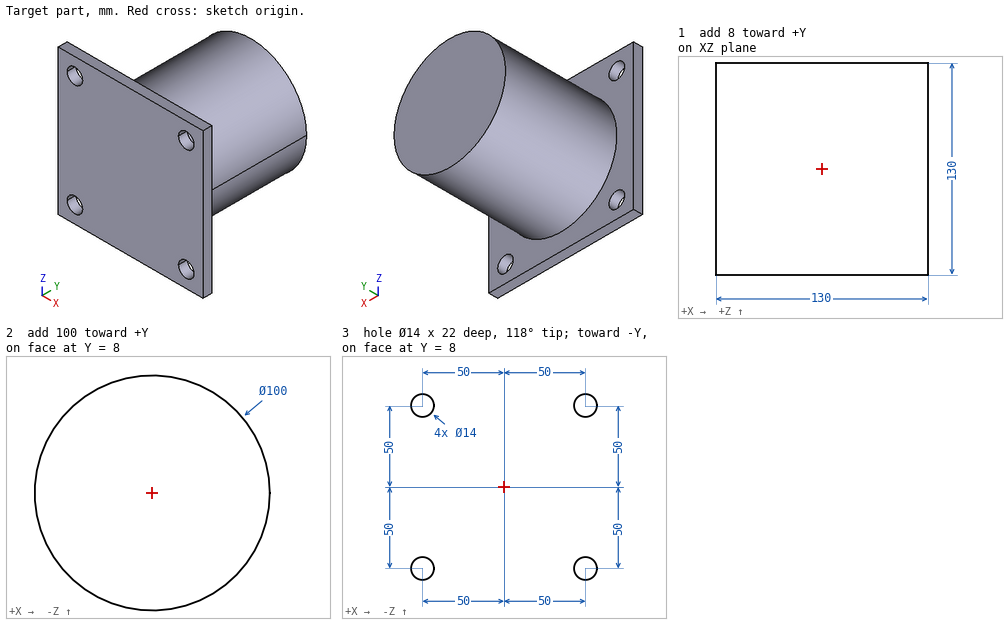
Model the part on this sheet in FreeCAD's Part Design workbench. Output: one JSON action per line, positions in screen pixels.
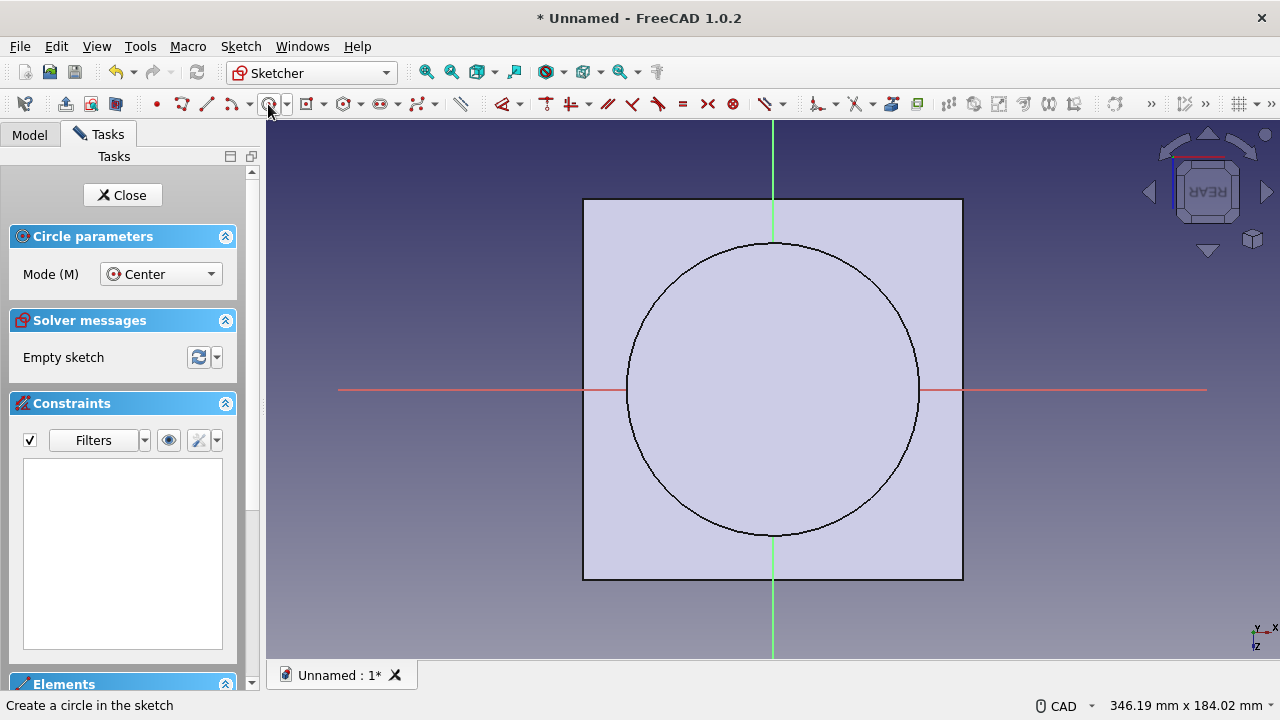
{"action": "left_click", "coordinate": [627, 243]}
{"action": "left_click", "coordinate": [641, 229]}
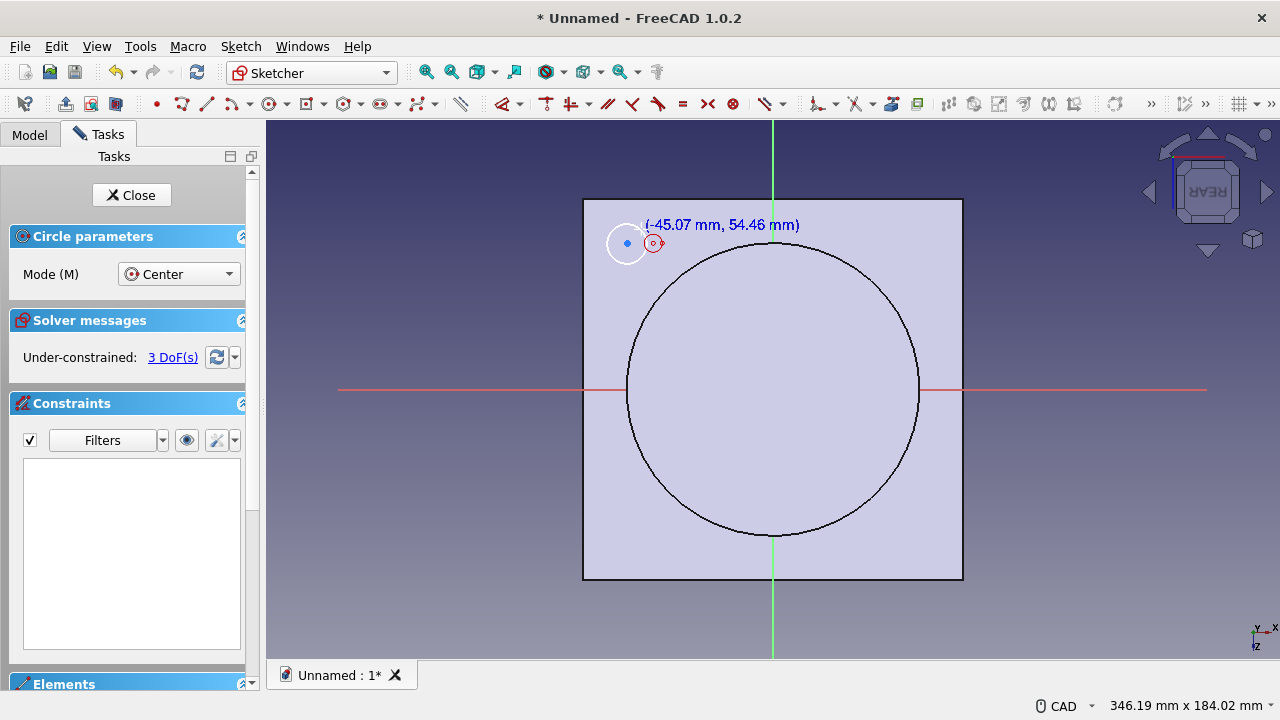
{"action": "left_click", "coordinate": [919, 243]}
{"action": "left_click", "coordinate": [934, 229]}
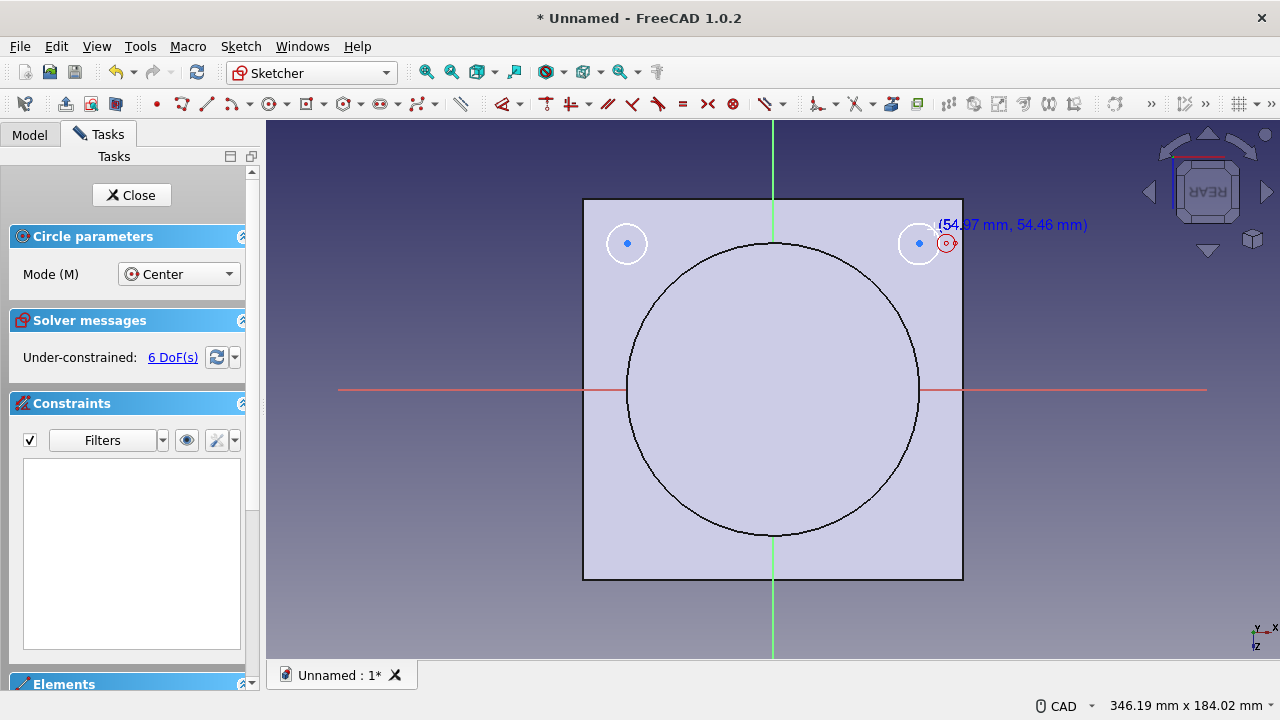
{"action": "left_click", "coordinate": [919, 536]}
{"action": "left_click", "coordinate": [934, 521]}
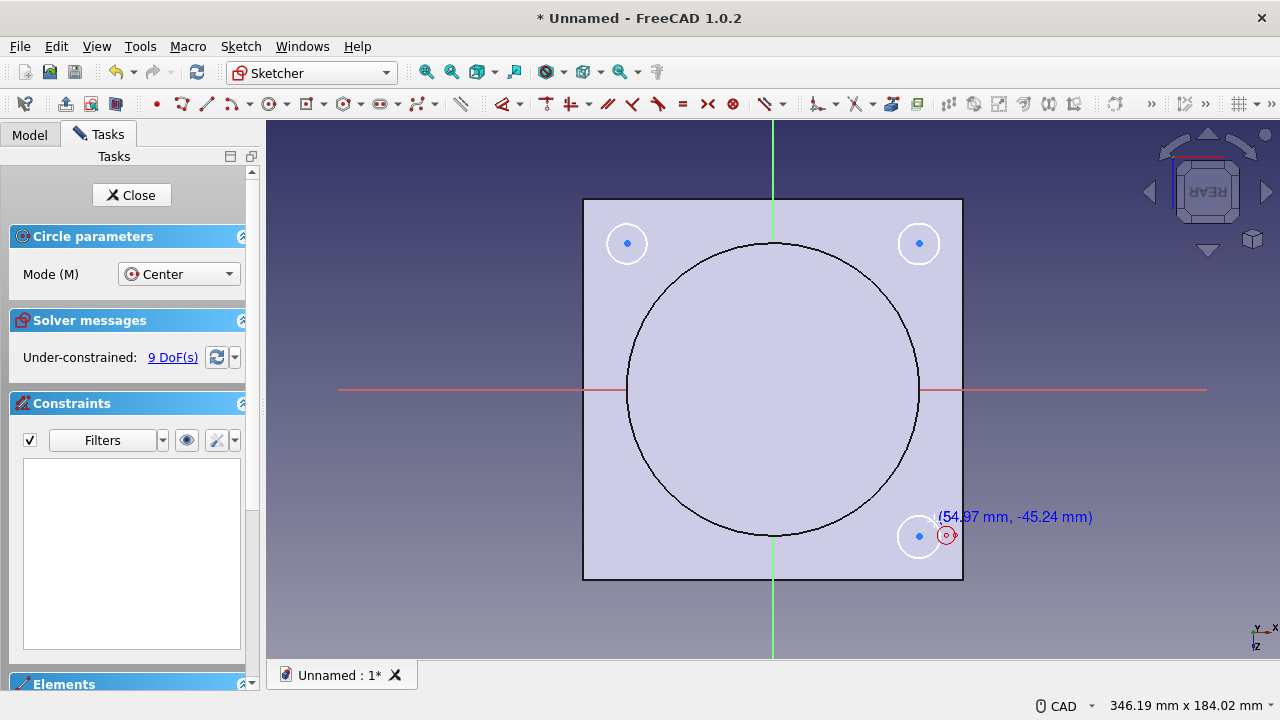
{"action": "left_click", "coordinate": [627, 536]}
{"action": "left_click", "coordinate": [641, 521]}
{"action": "key", "text": "Escape"}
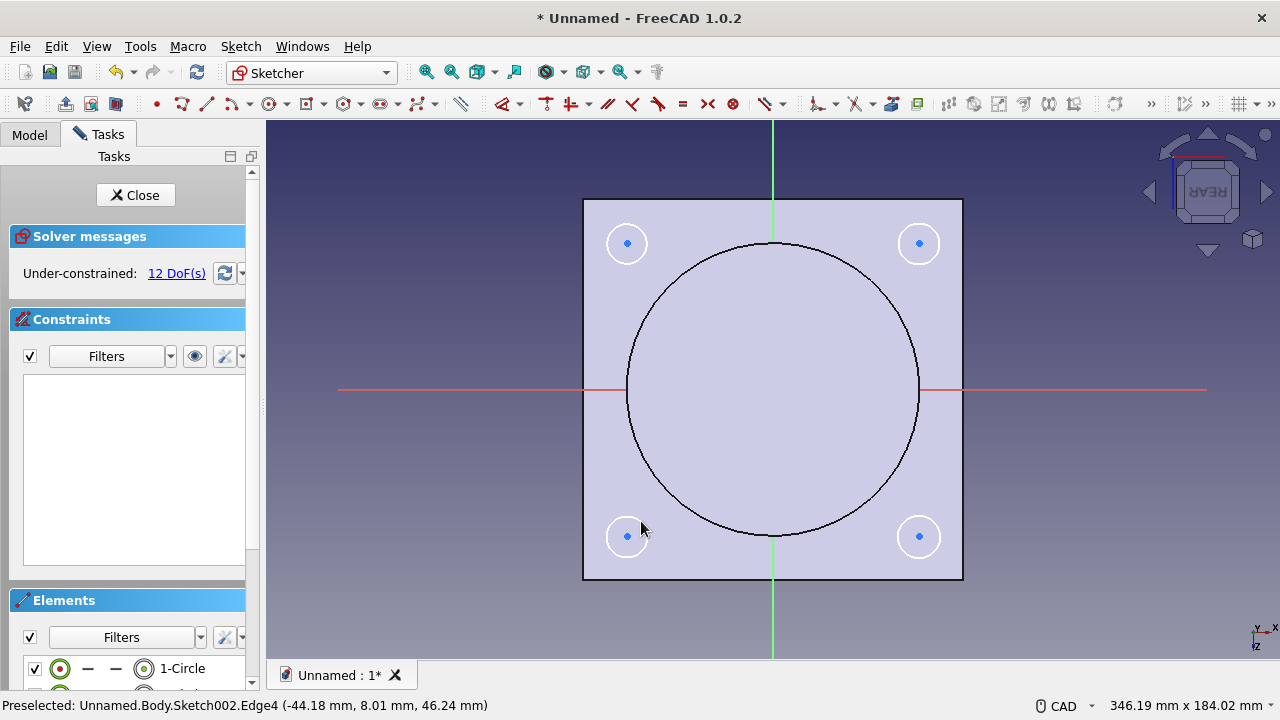
{"action": "left_click", "coordinate": [641, 230]}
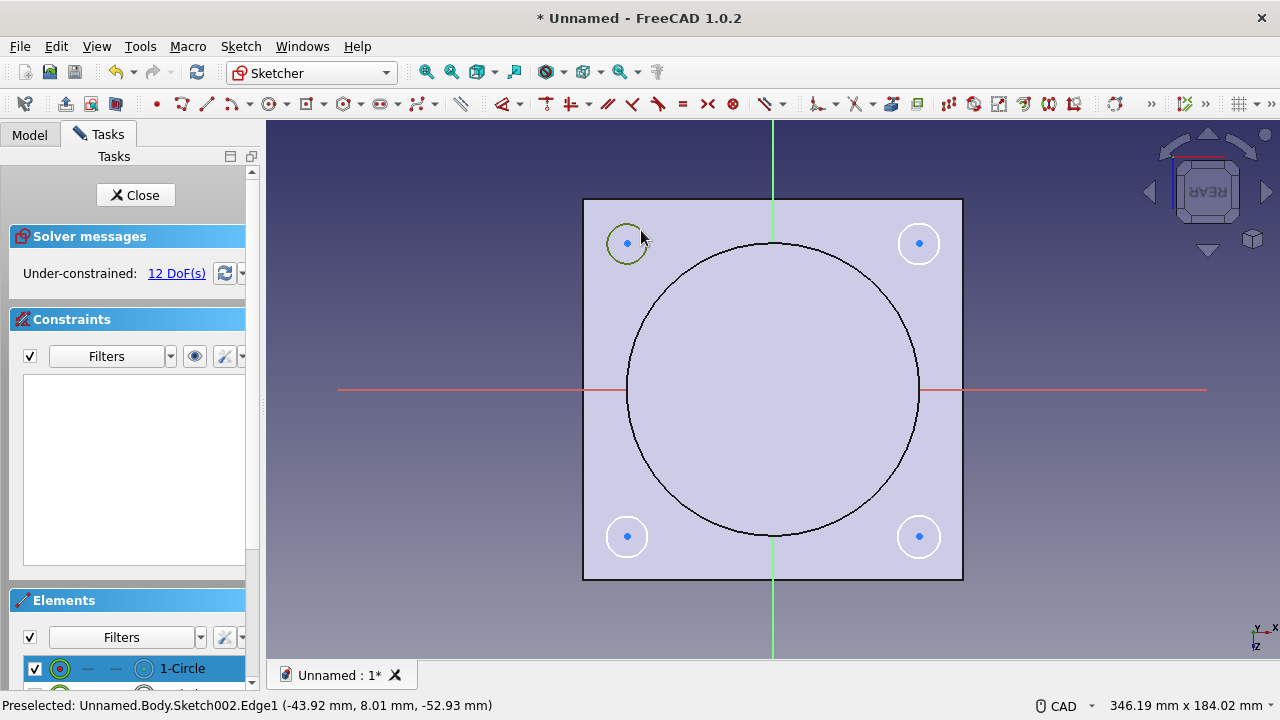
{"action": "left_click", "coordinate": [933, 229]}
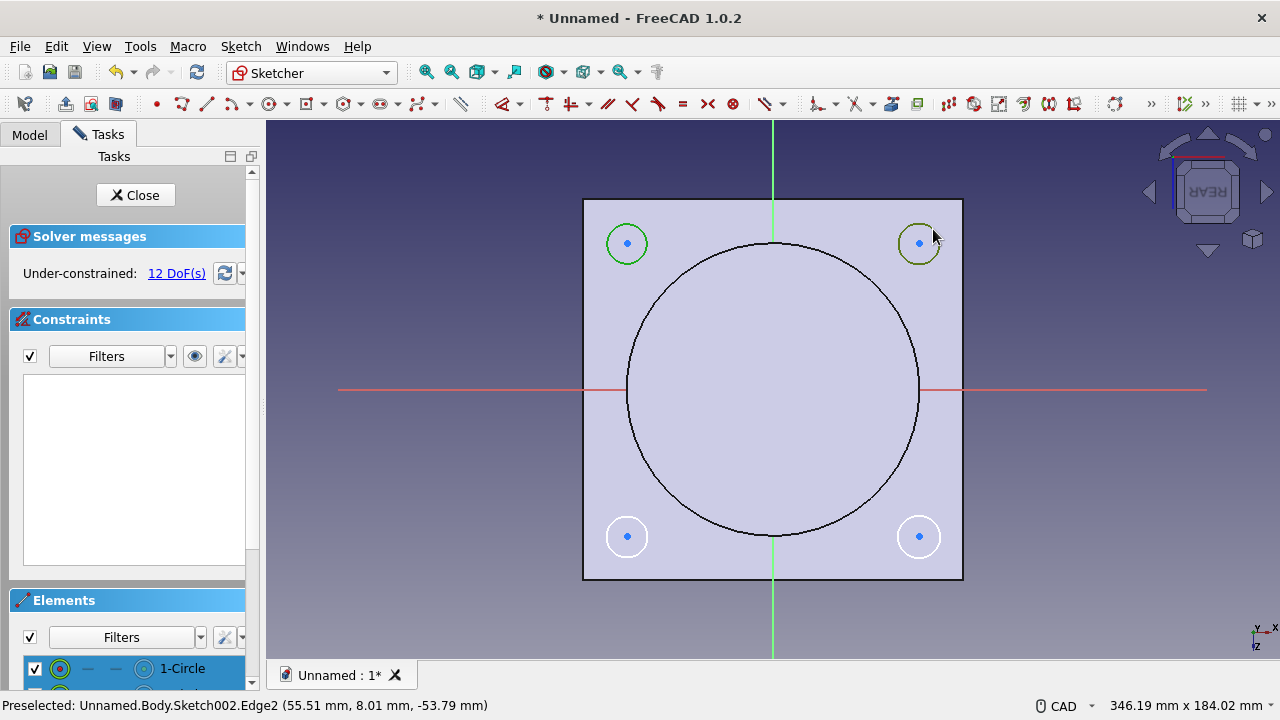
{"action": "left_click", "coordinate": [934, 522]}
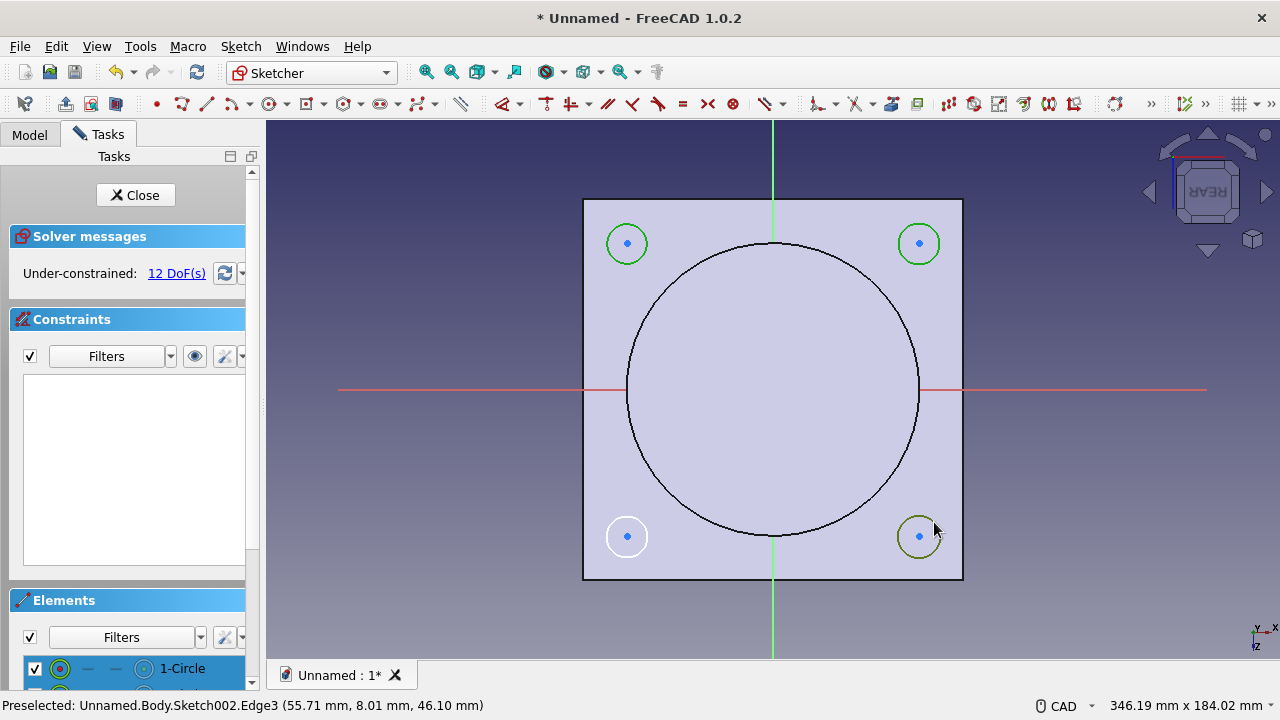
{"action": "left_click", "coordinate": [641, 522]}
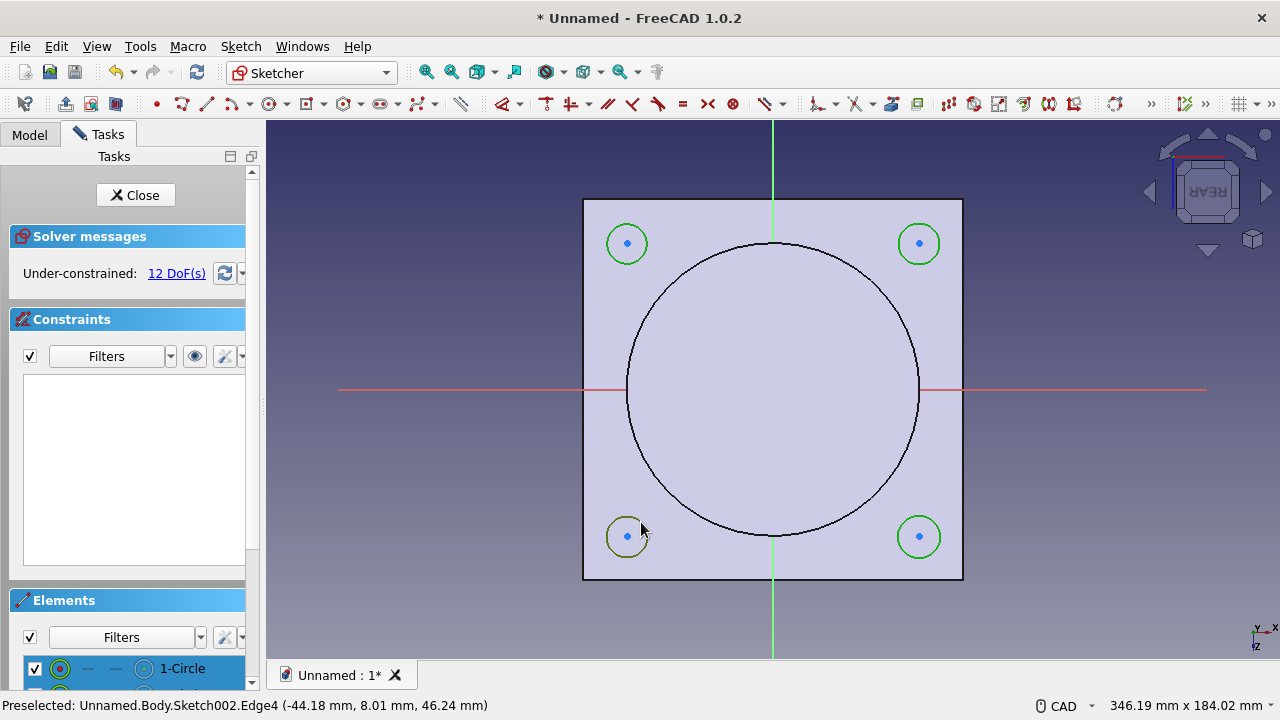
{"action": "left_click", "coordinate": [683, 104]}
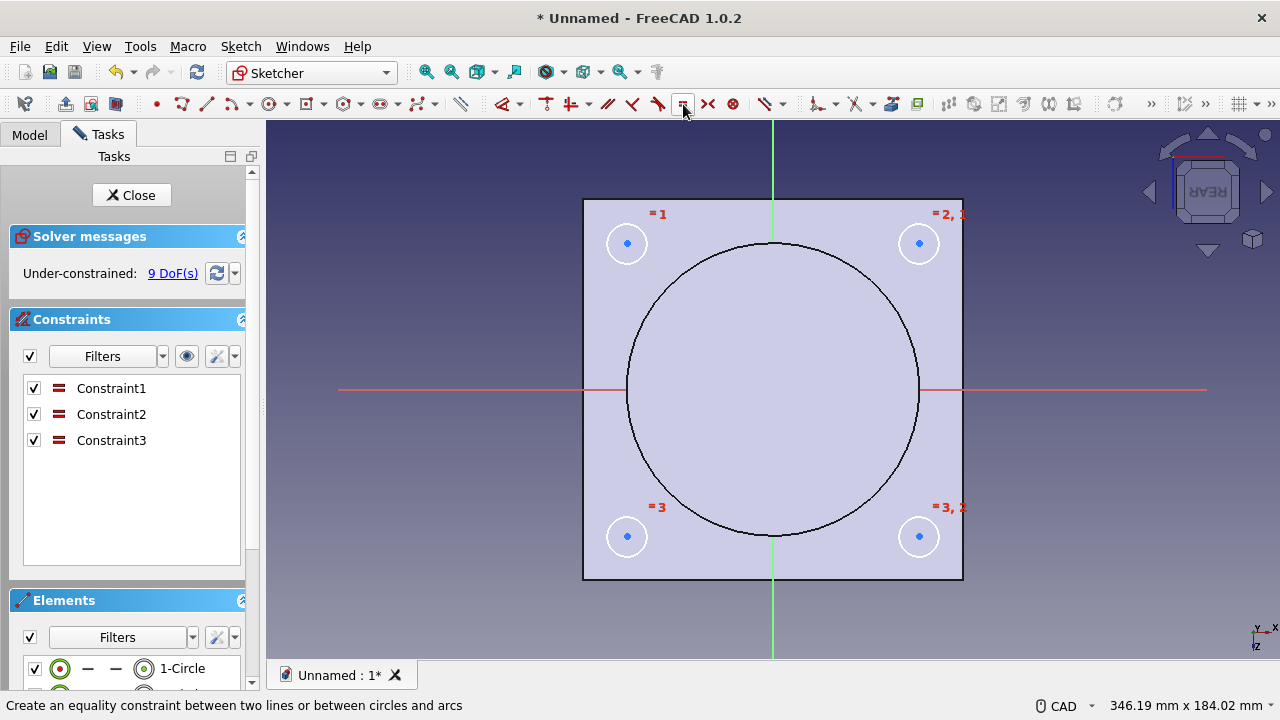
{"action": "key", "text": "d"}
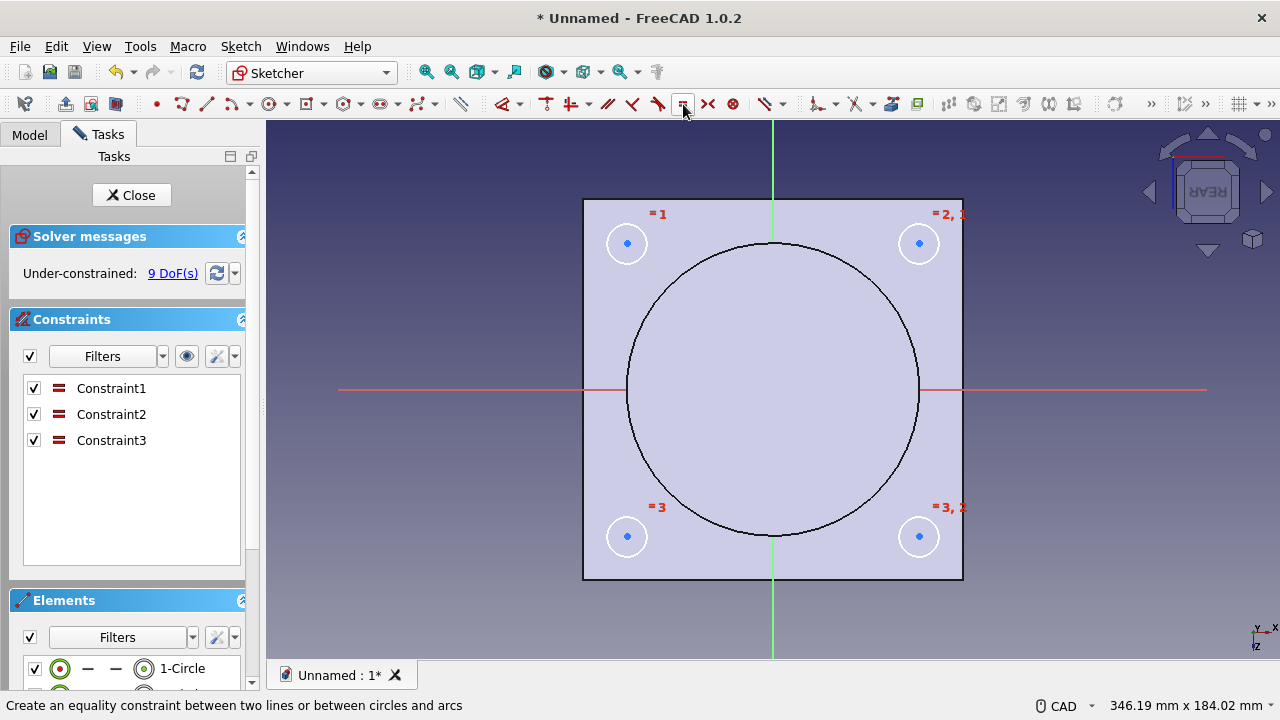
{"action": "left_click", "coordinate": [641, 230]}
{"action": "left_click", "coordinate": [664, 207]}